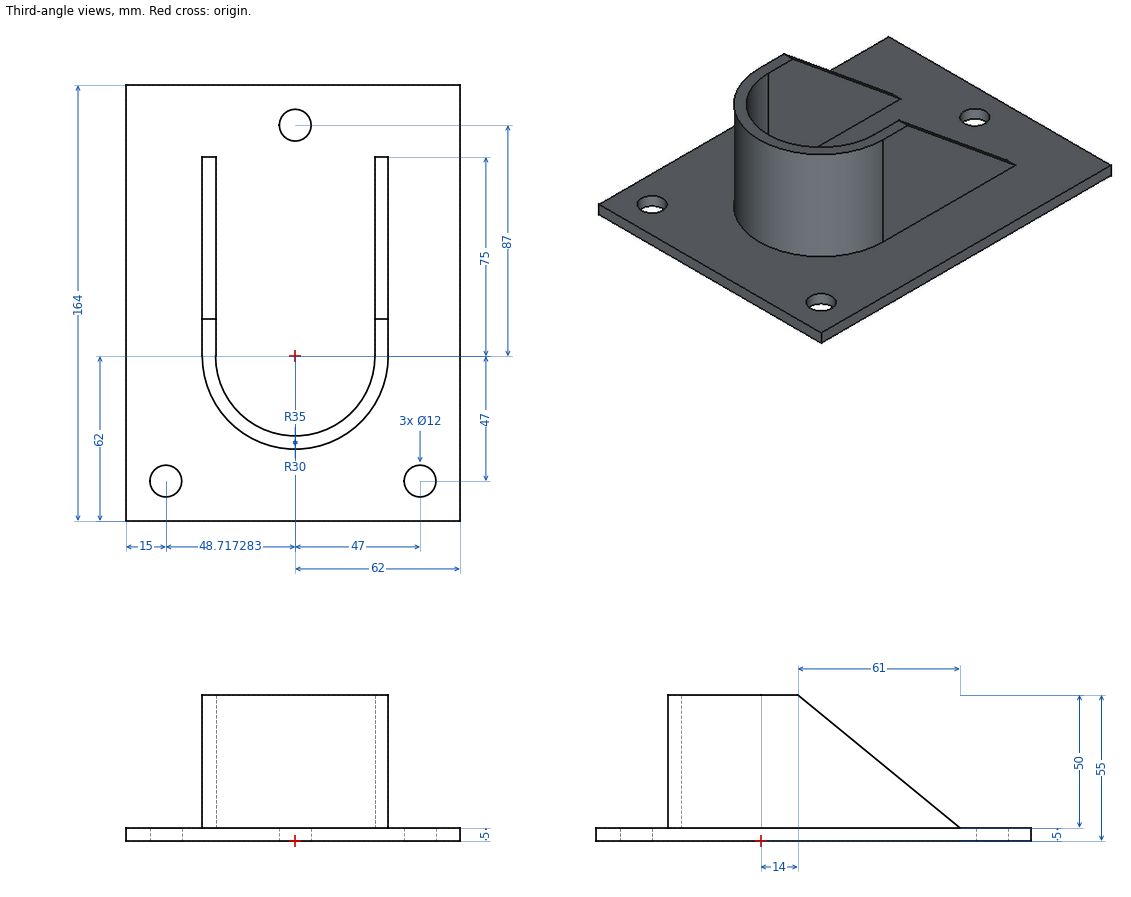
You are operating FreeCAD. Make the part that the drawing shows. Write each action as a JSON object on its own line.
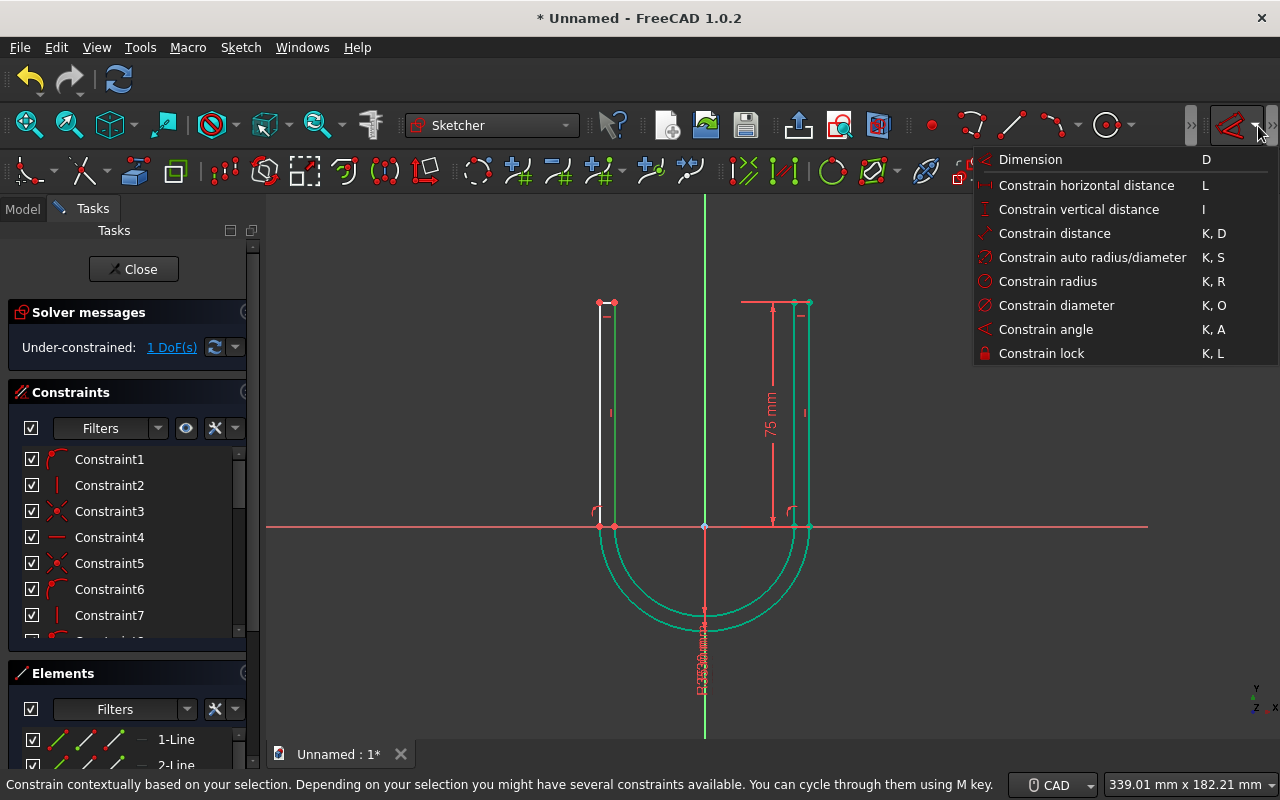
{"action": "left_click", "coordinate": [1126, 209]}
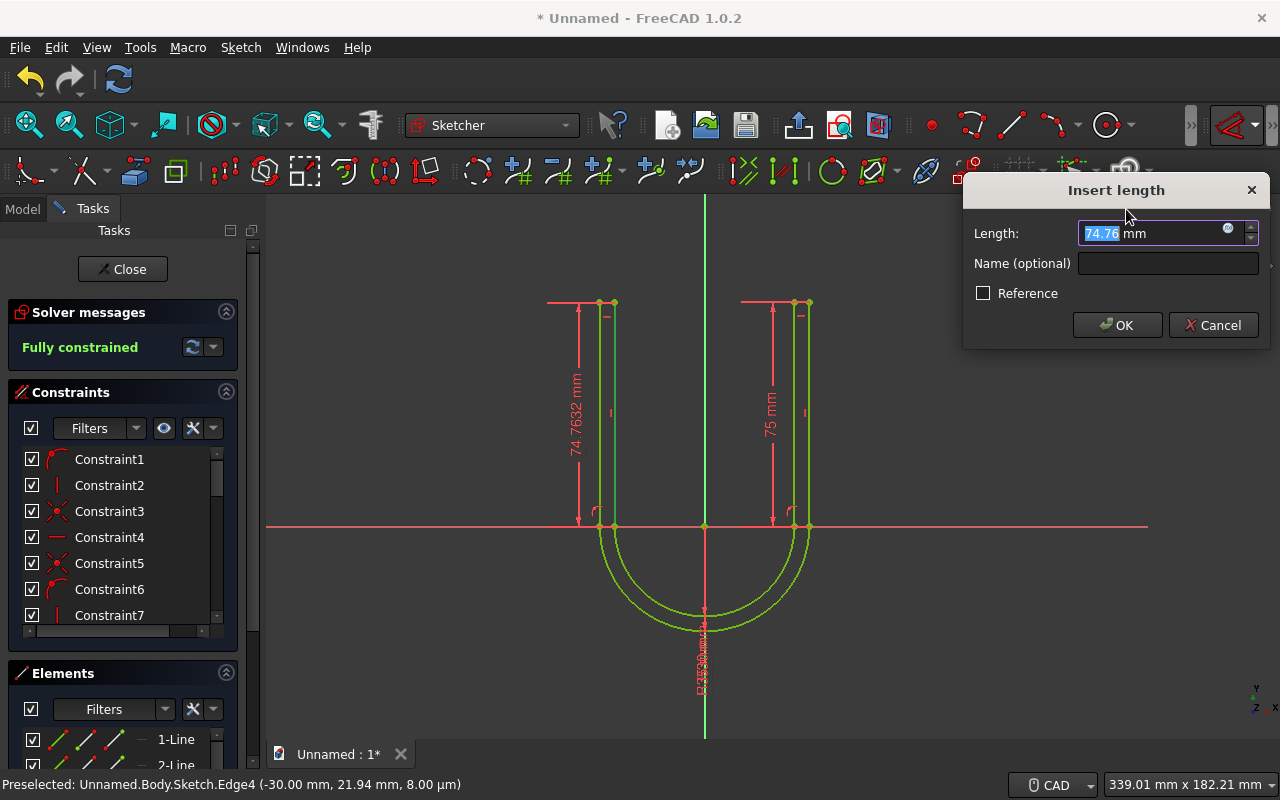
{"action": "type", "text": "75"}
{"action": "key", "text": "Return"}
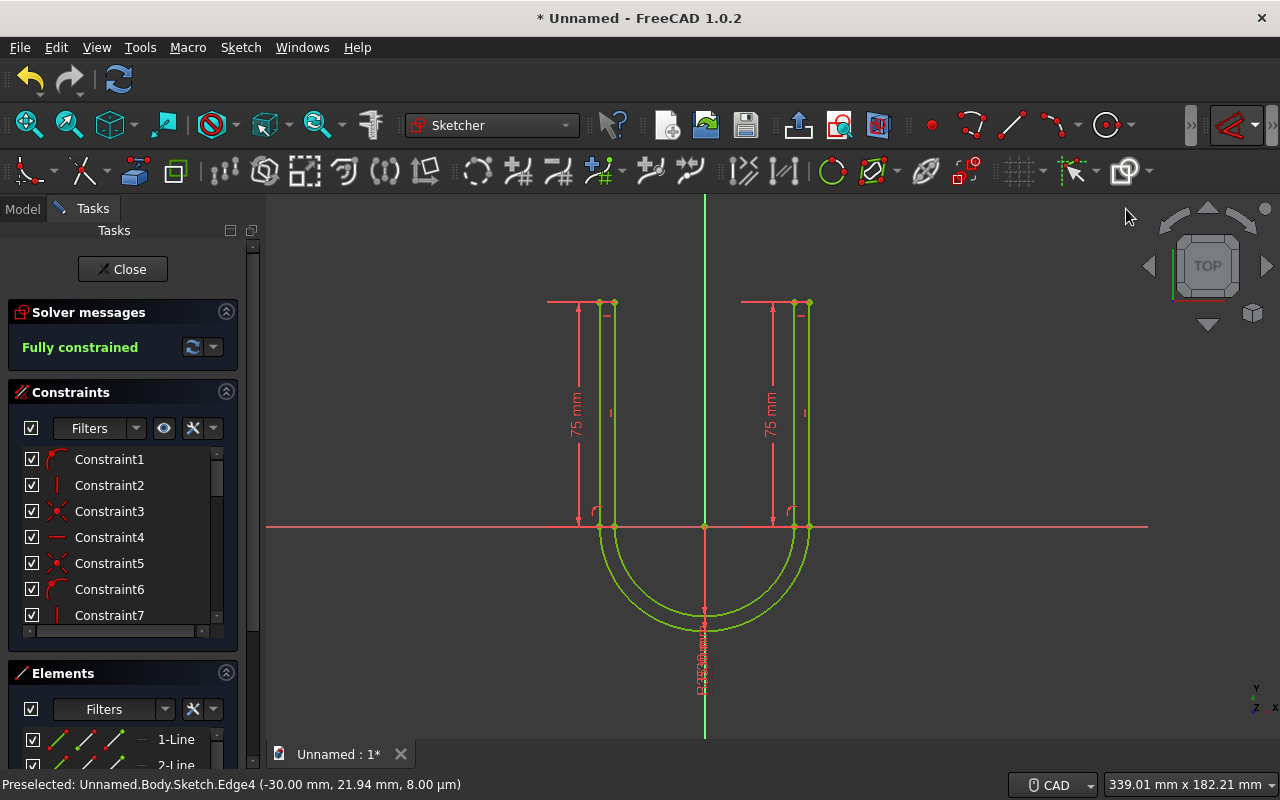
{"action": "left_click", "coordinate": [123, 269]}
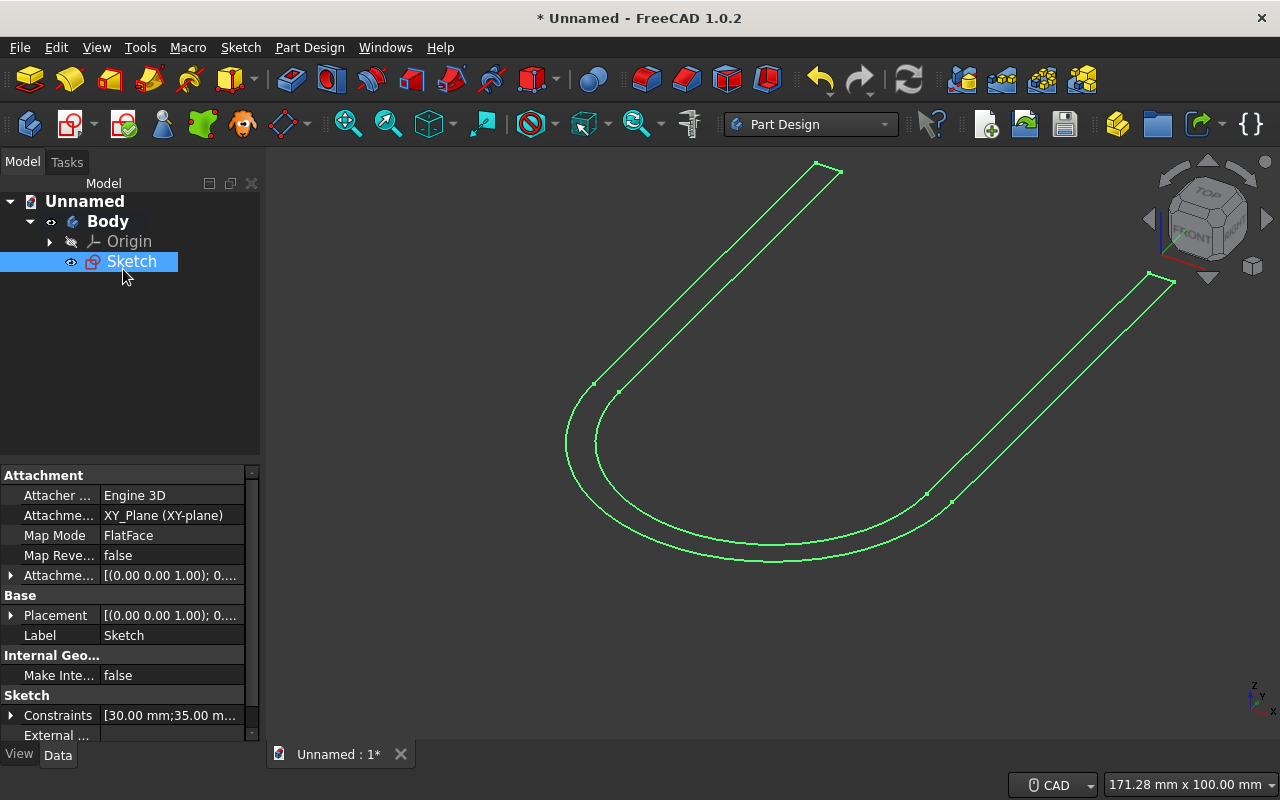
{"action": "left_click", "coordinate": [30, 80]}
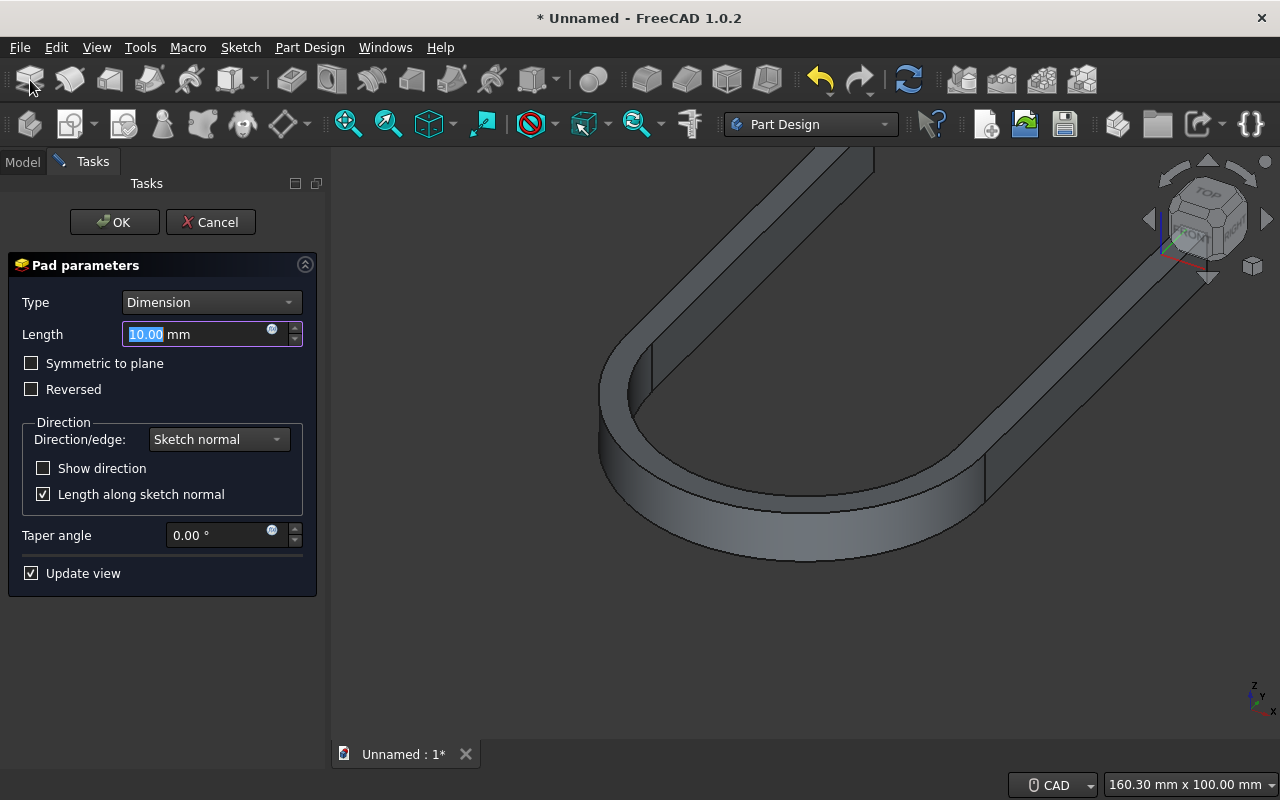
{"action": "type", "text": "55"}
{"action": "key", "text": "Tab"}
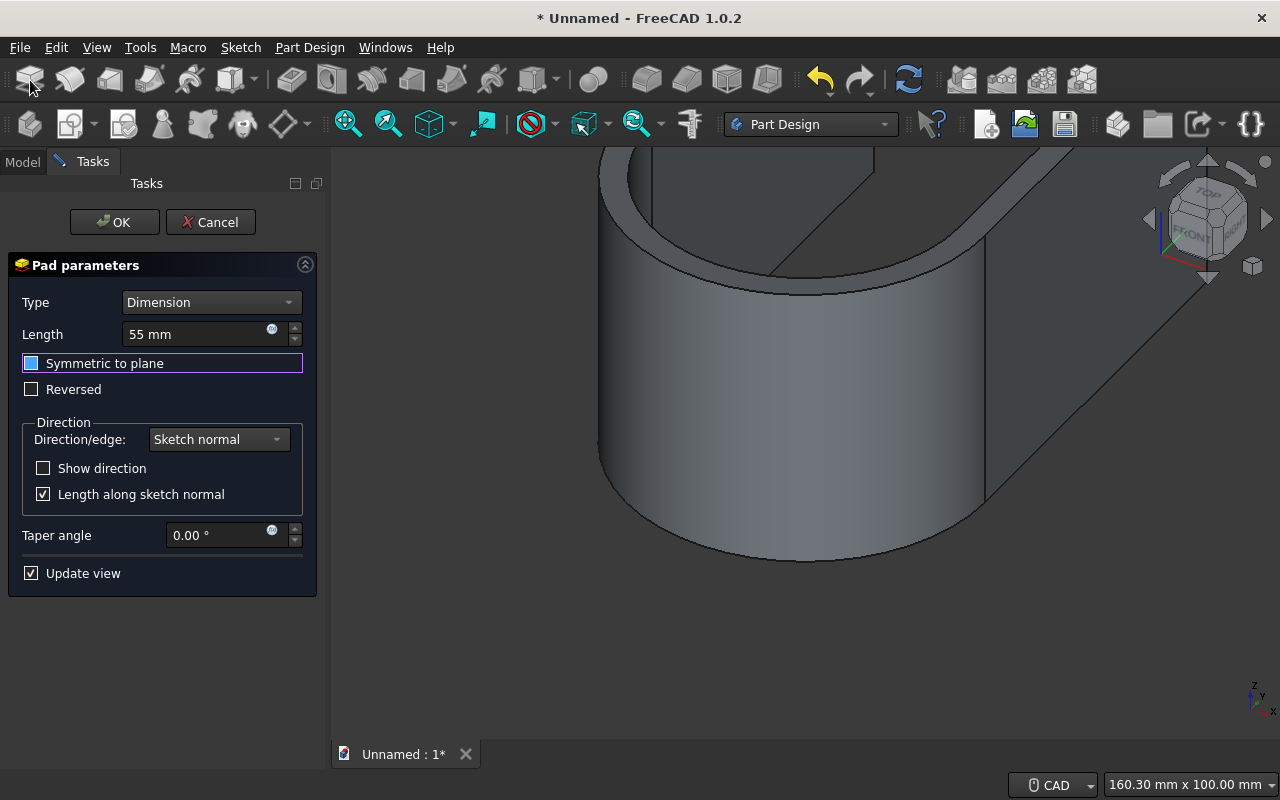
{"action": "left_click", "coordinate": [115, 222]}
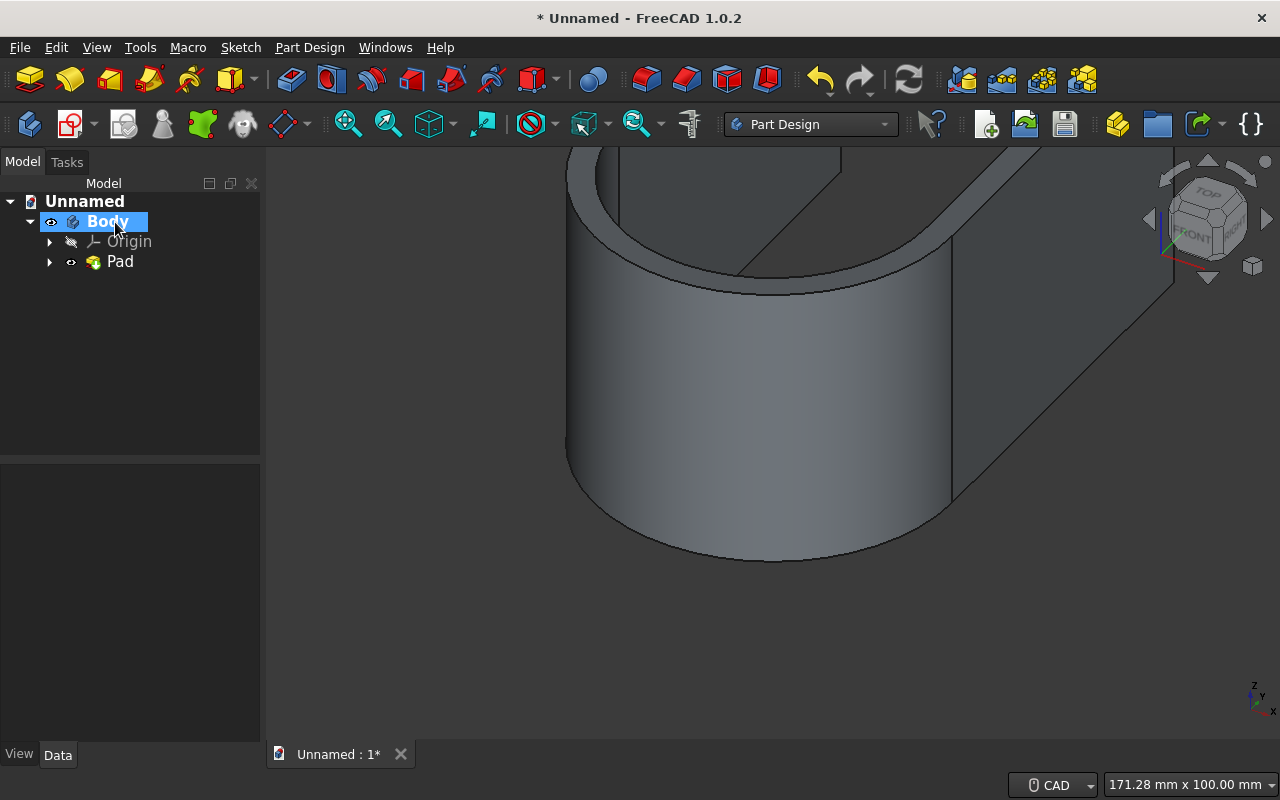
{"action": "left_click", "coordinate": [350, 124]}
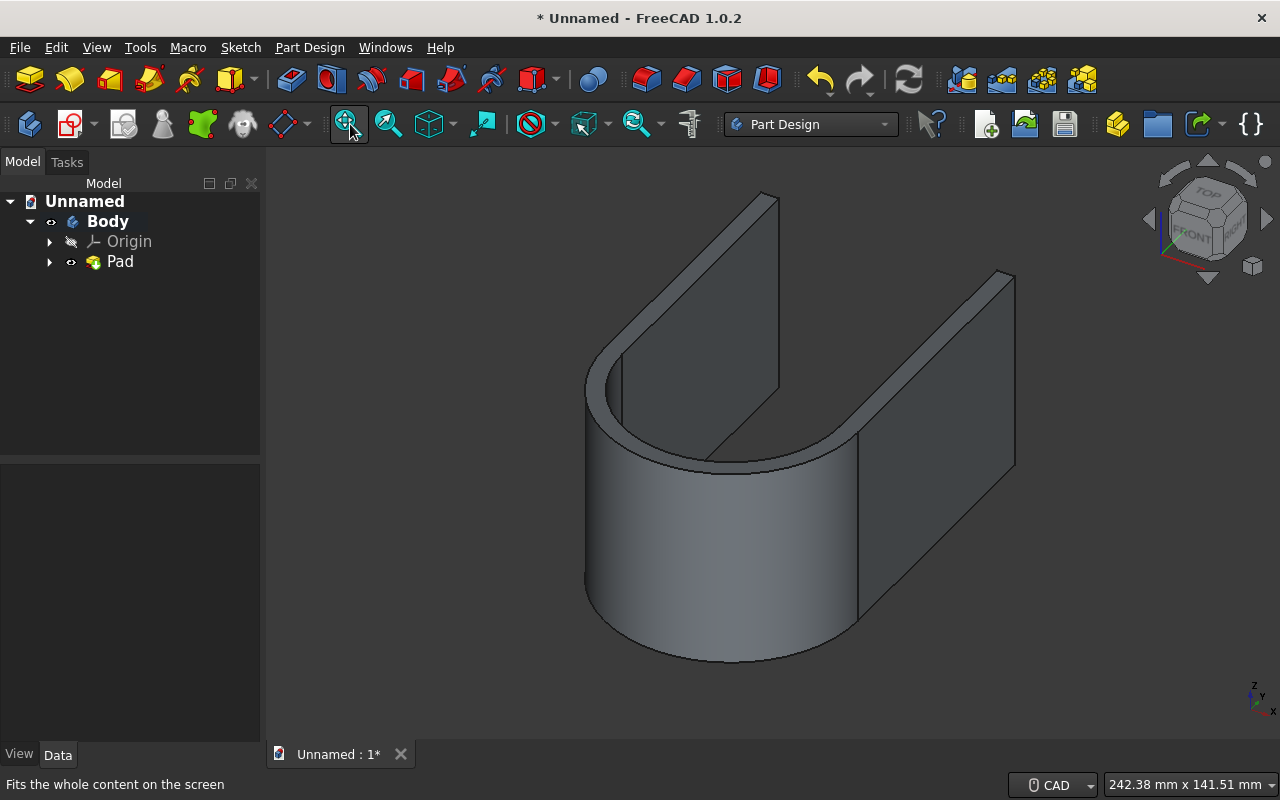
{"action": "left_click", "coordinate": [70, 124]}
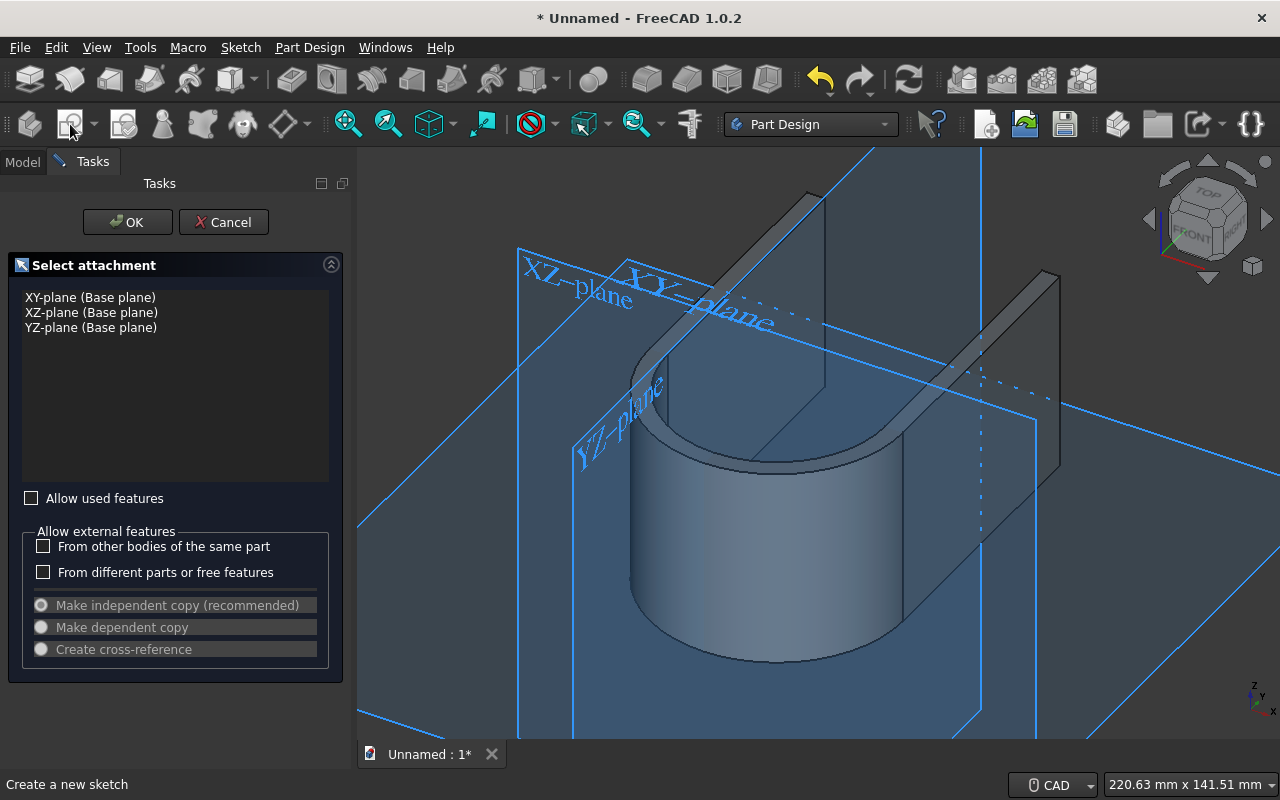
{"action": "left_click", "coordinate": [82, 298]}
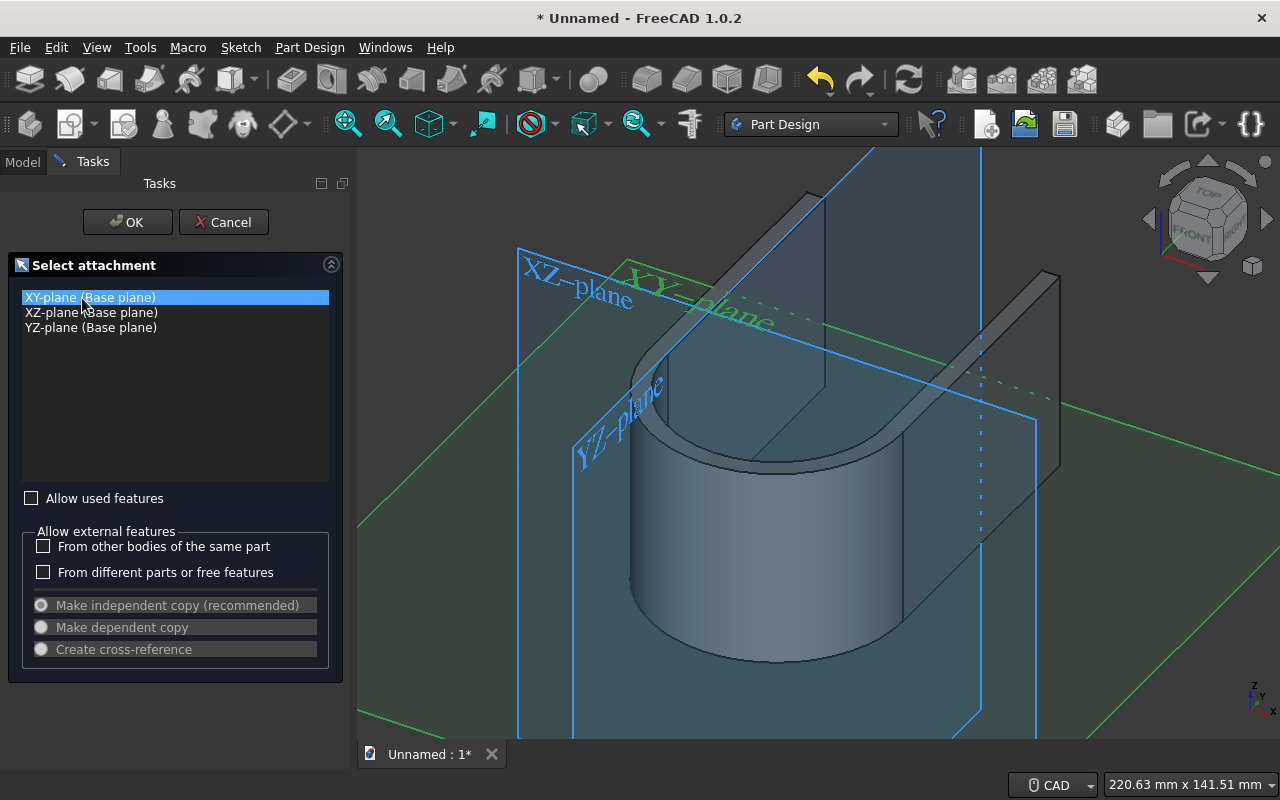
{"action": "left_click", "coordinate": [128, 222]}